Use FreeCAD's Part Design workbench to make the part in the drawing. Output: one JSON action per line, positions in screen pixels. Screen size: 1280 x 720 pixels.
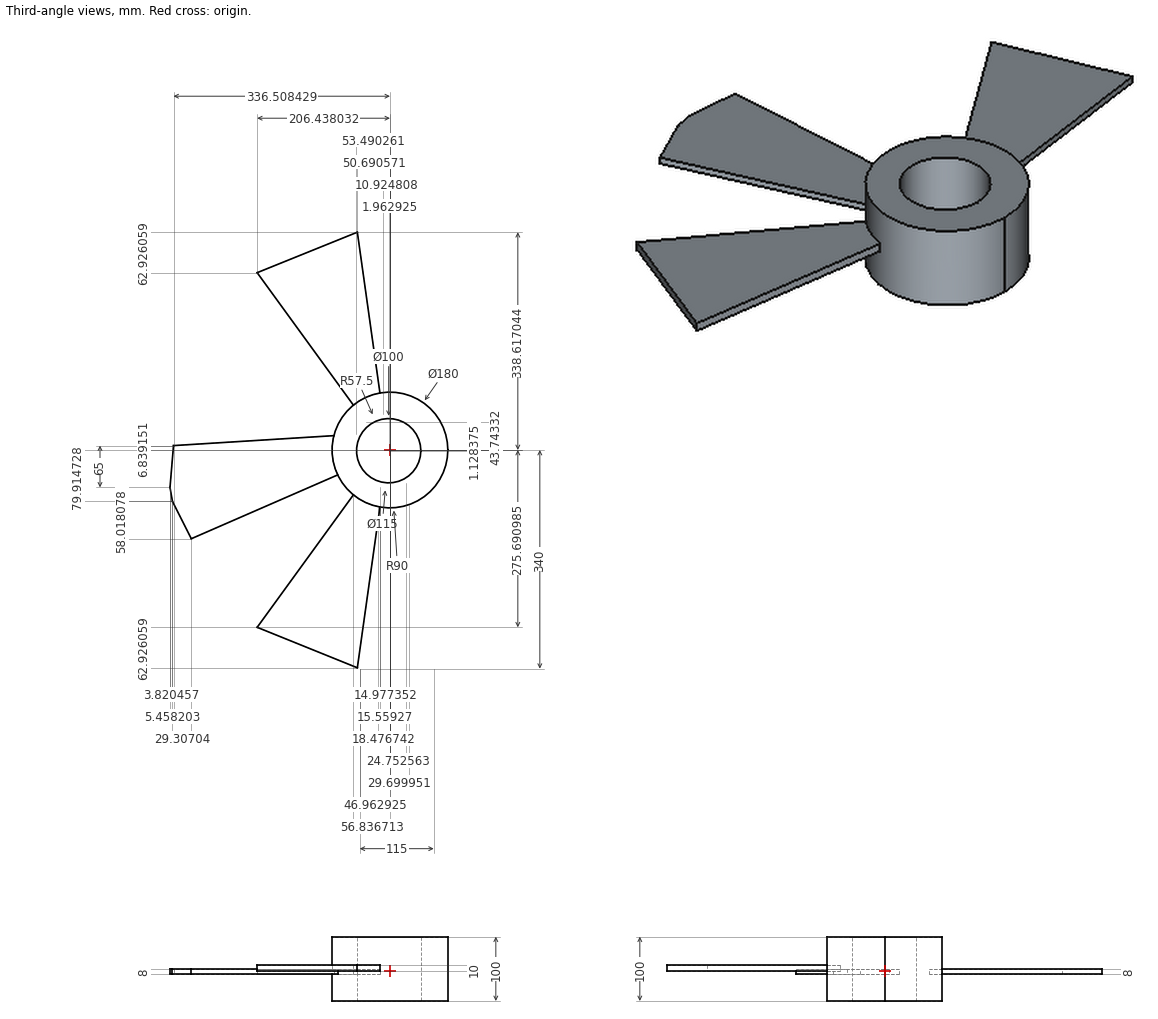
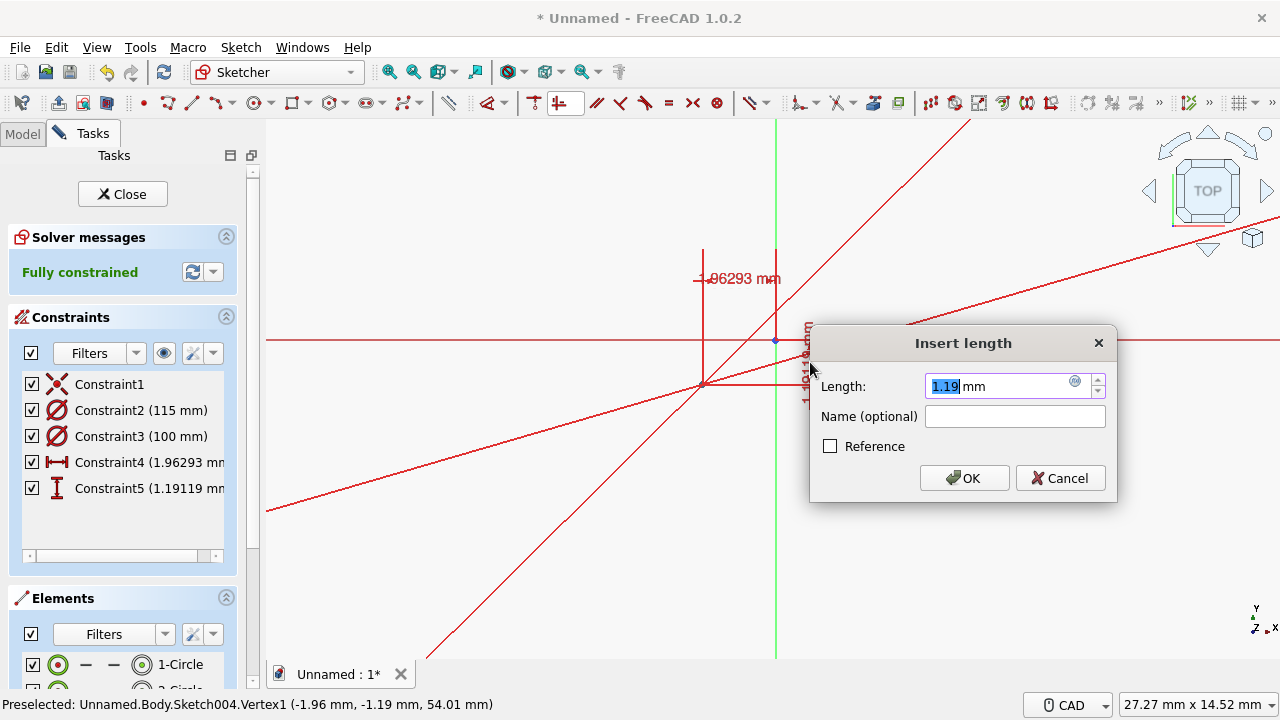
{"action": "type", "text": "1.128375"}
{"action": "key", "text": "Return"}
{"action": "key", "text": "Escape"}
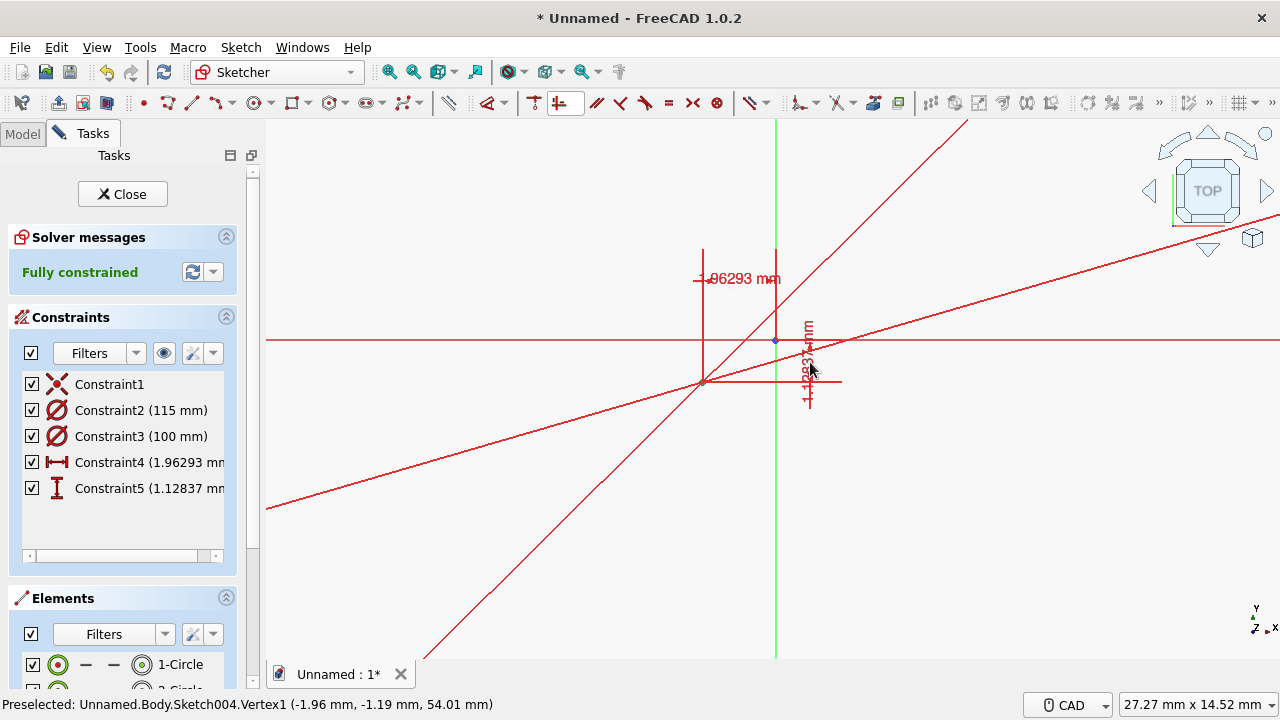
{"action": "left_click", "coordinate": [123, 194]}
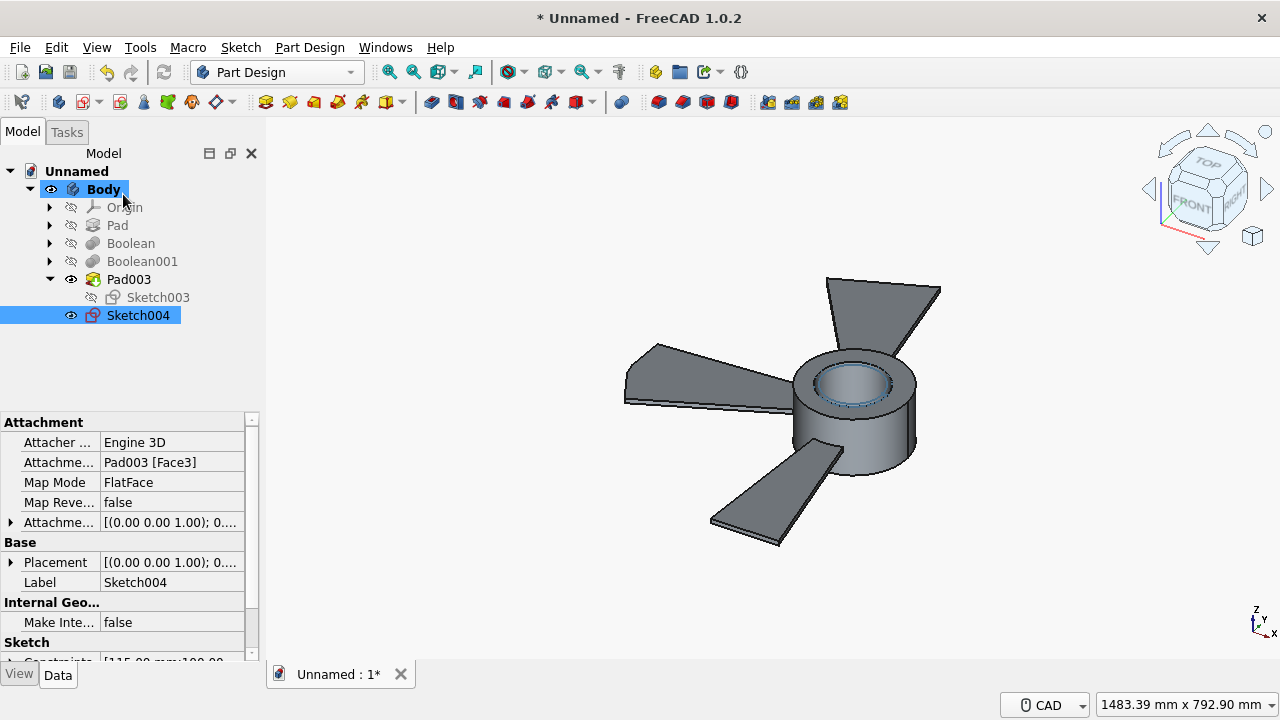
{"action": "left_click", "coordinate": [266, 102]}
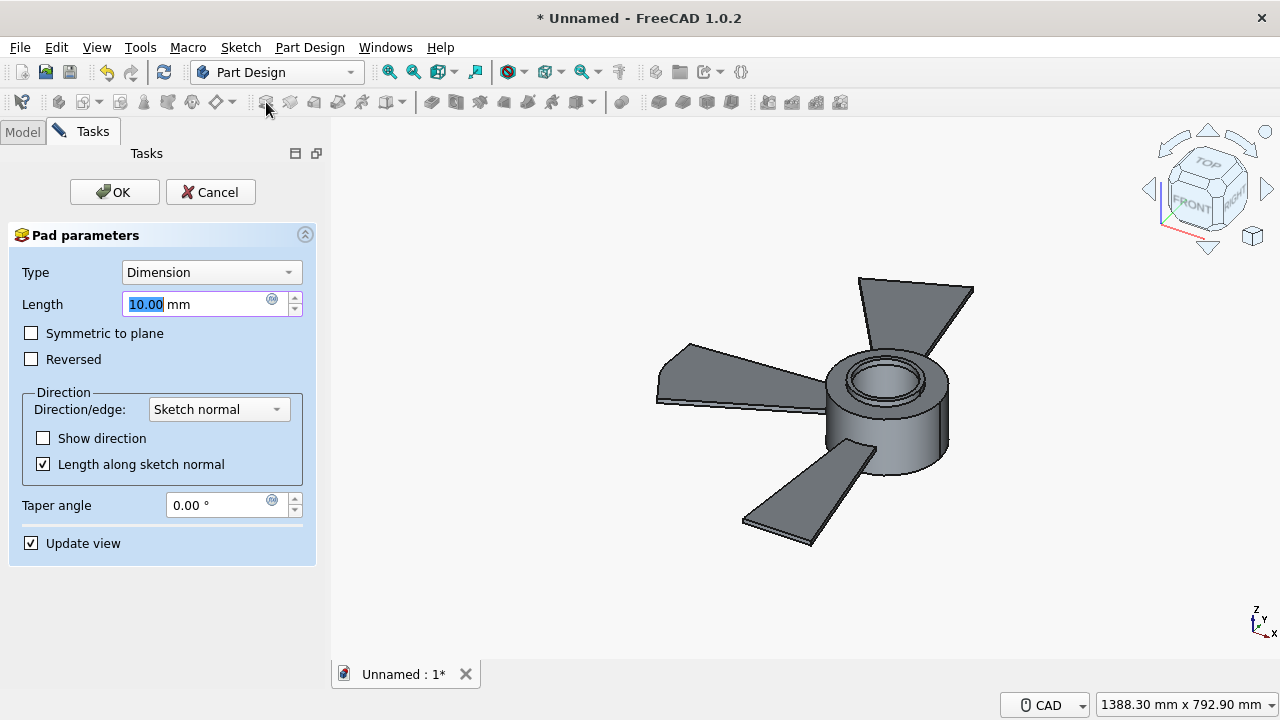
{"action": "type", "text": "100"}
{"action": "key", "text": "Tab"}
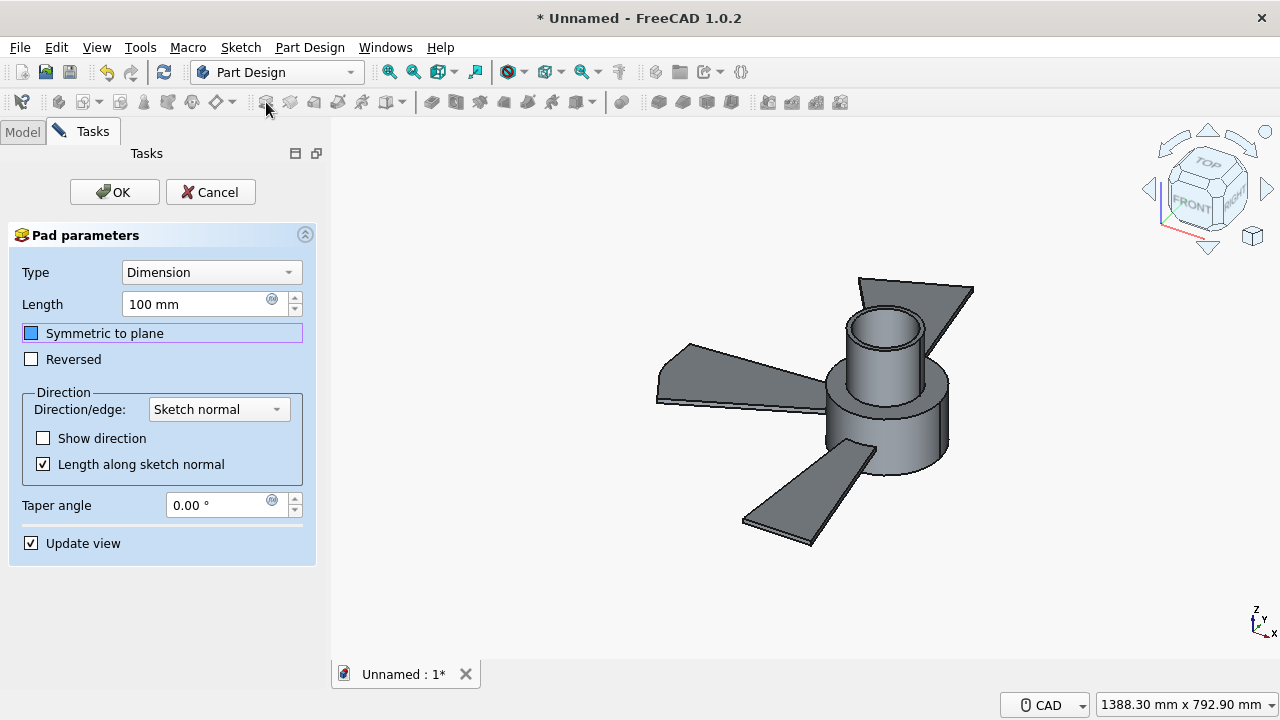
{"action": "left_click", "coordinate": [30, 359]}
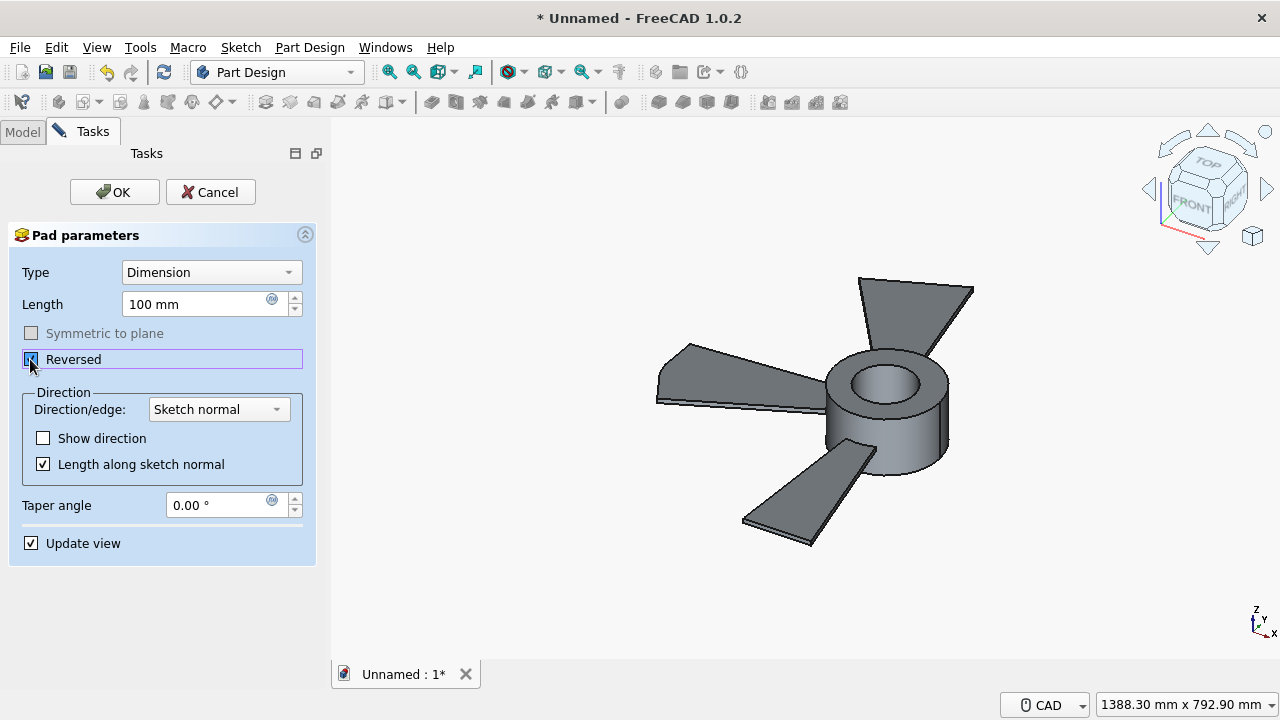
{"action": "left_click", "coordinate": [115, 192]}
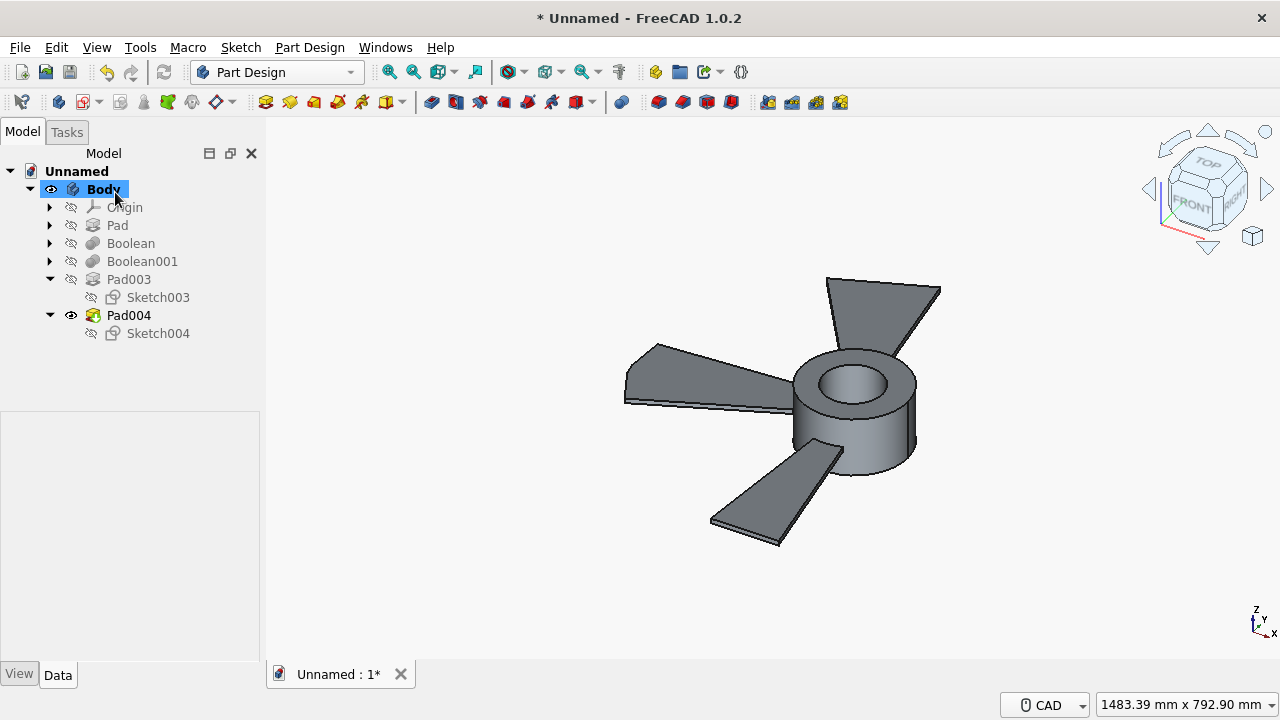
{"action": "left_click", "coordinate": [666, 375]}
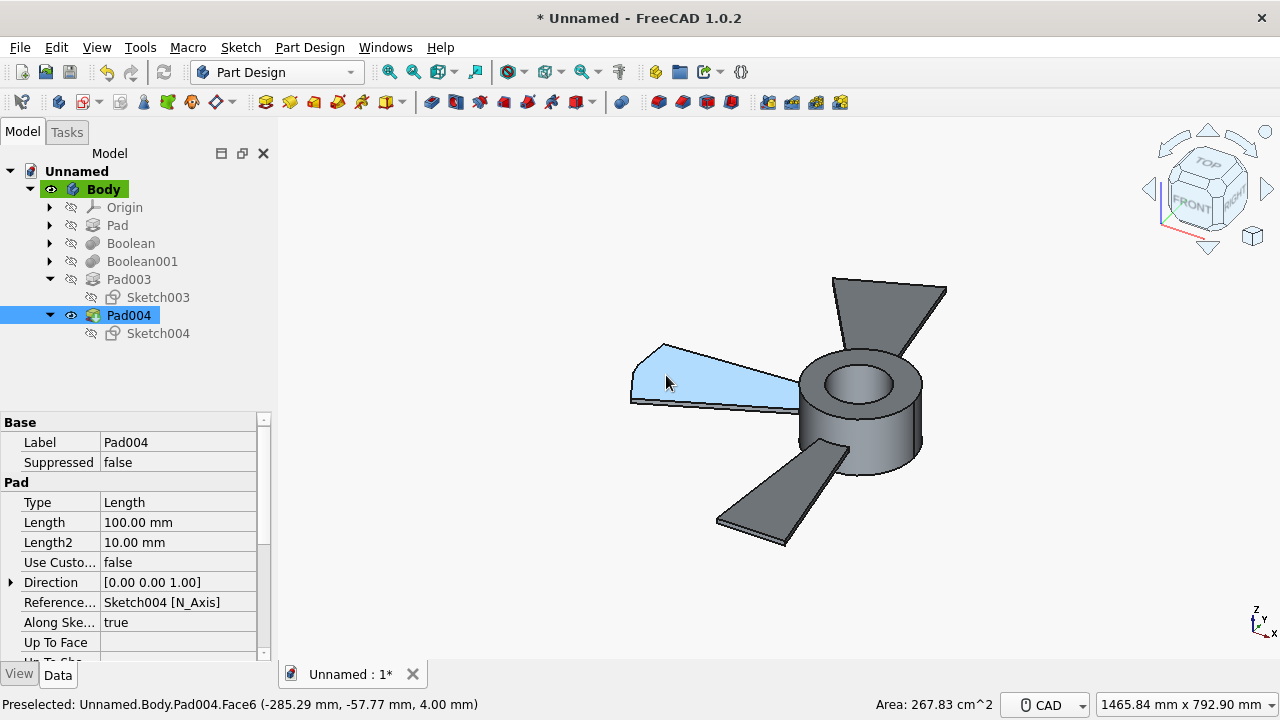
{"action": "left_click", "coordinate": [84, 102]}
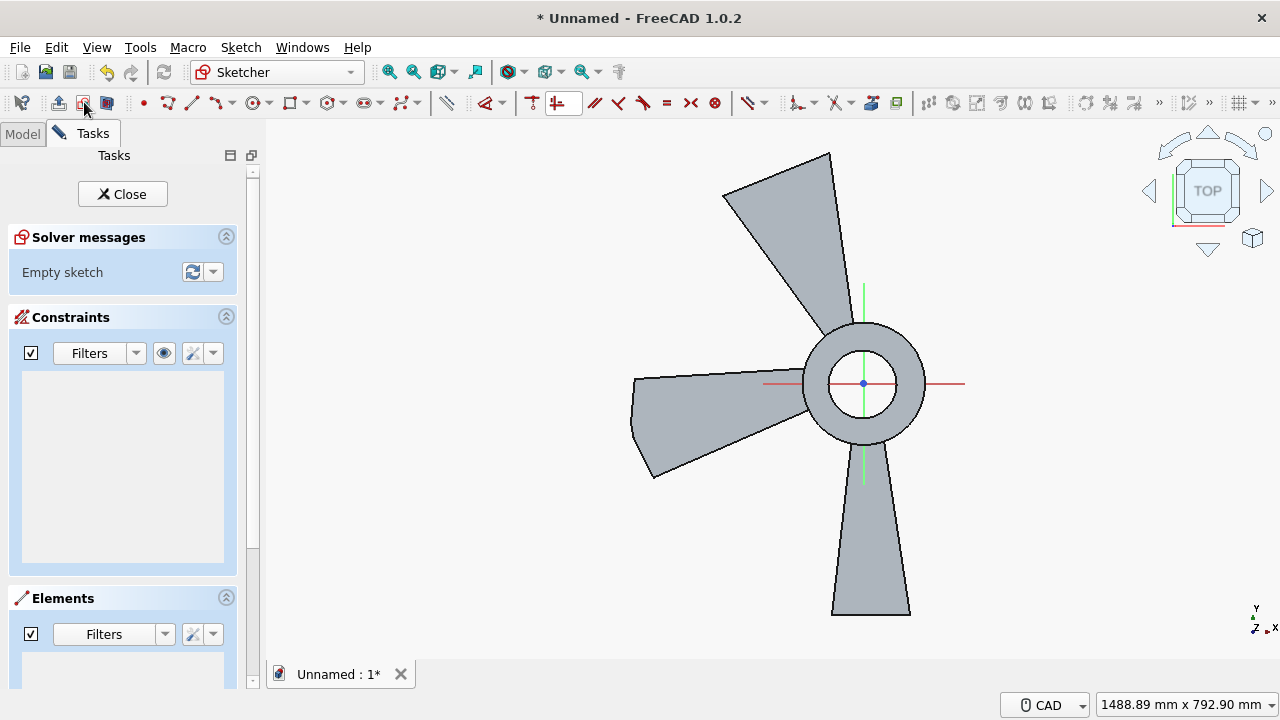
{"action": "scroll", "coordinate": [294, 147], "scroll_direction": "down", "scroll_amount": 1}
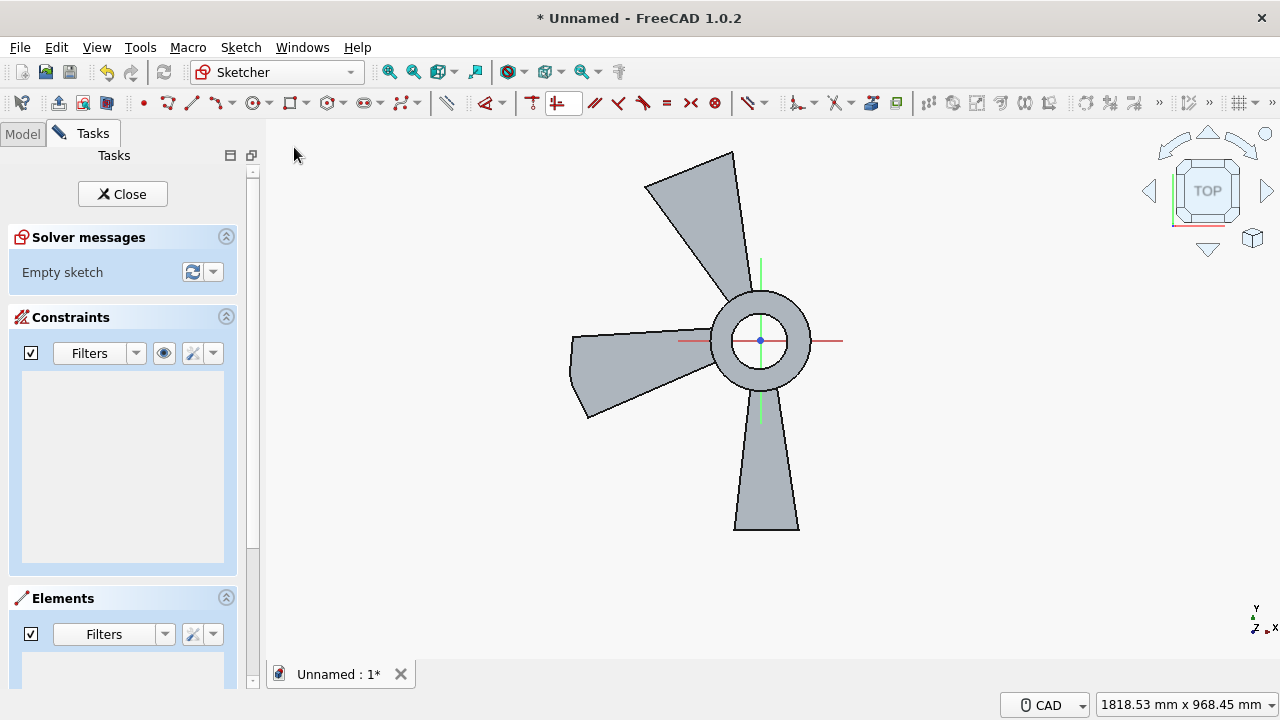
{"action": "scroll", "coordinate": [842, 492], "scroll_direction": "up", "scroll_amount": 3}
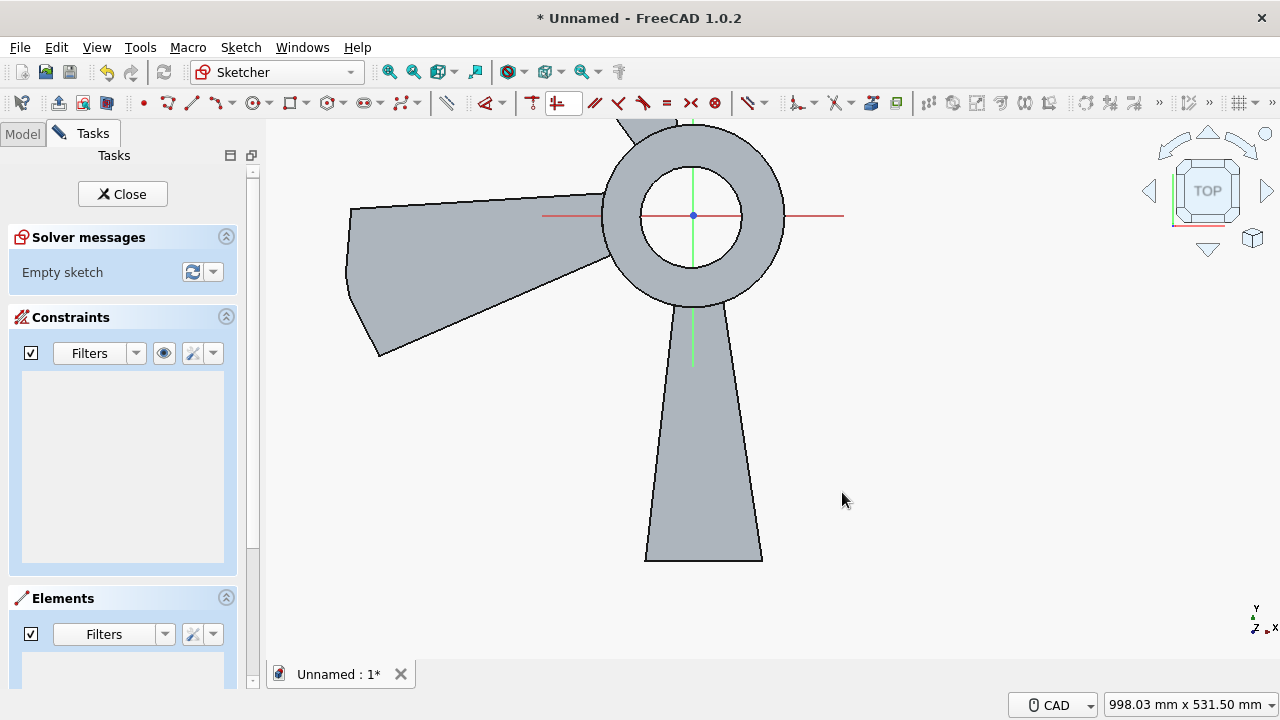
{"action": "left_click", "coordinate": [168, 104]}